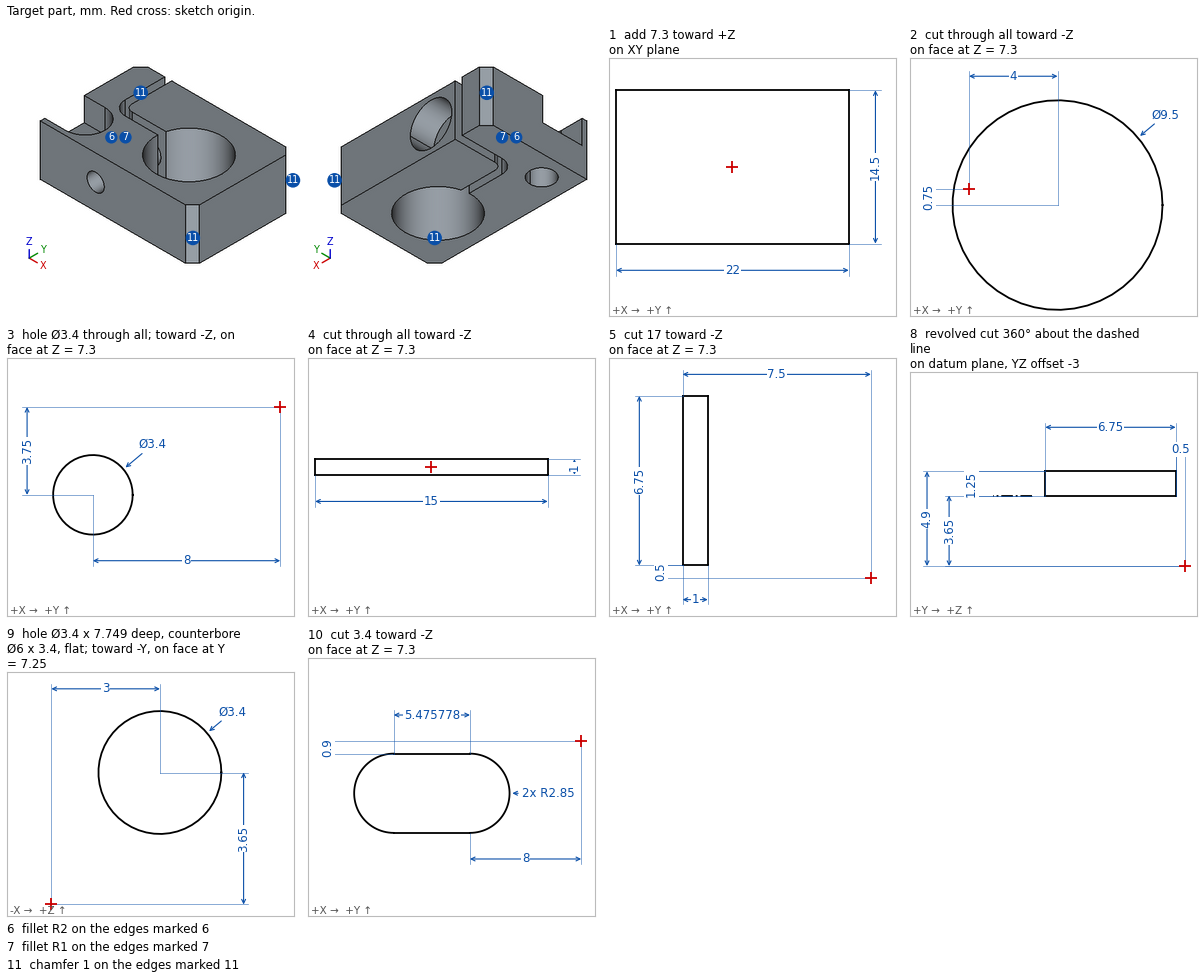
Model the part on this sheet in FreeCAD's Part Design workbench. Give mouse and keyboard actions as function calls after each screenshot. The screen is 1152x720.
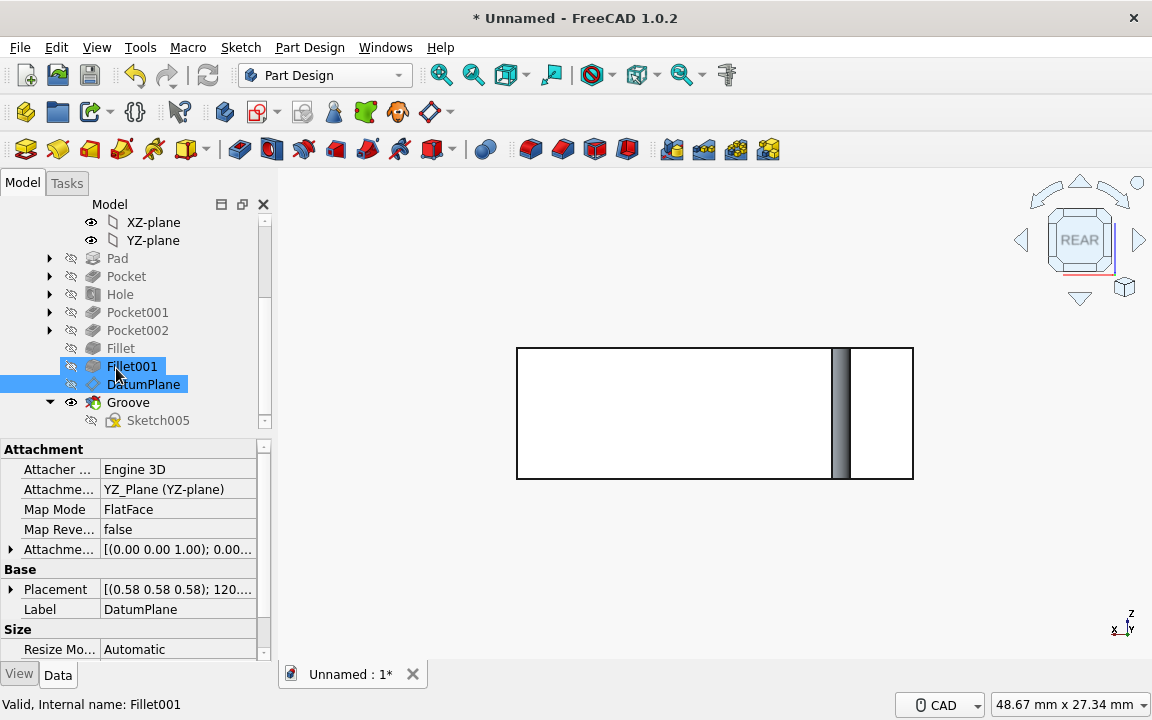
click(585, 412)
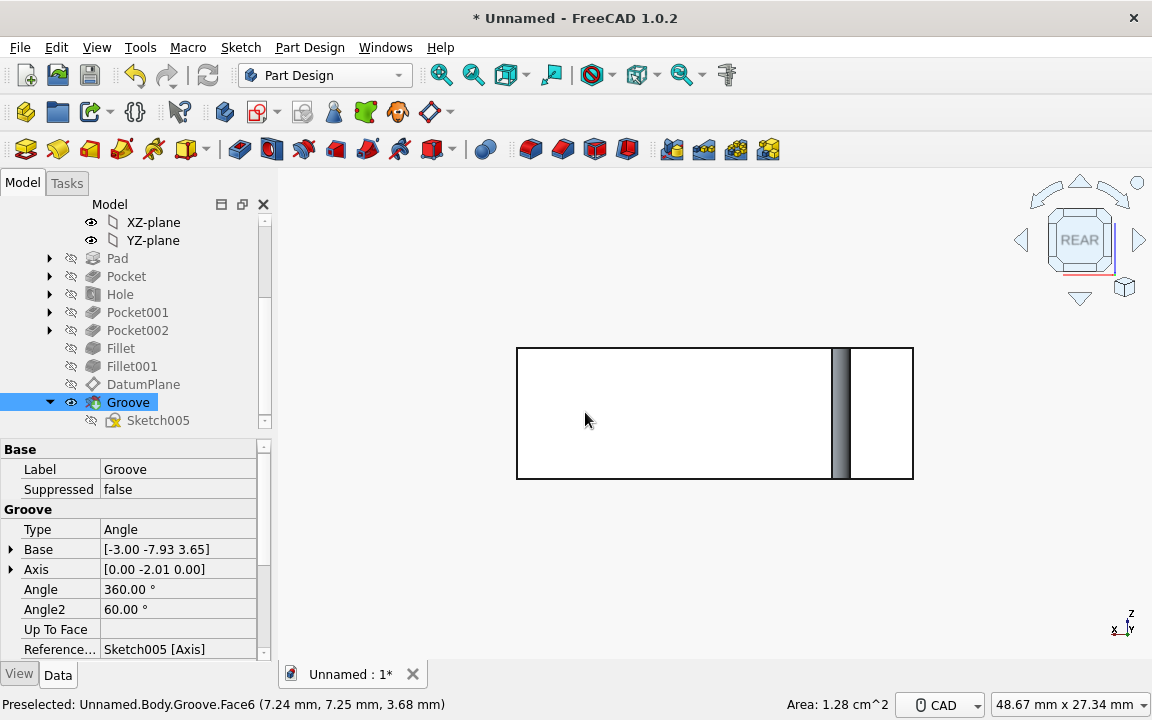
click(258, 112)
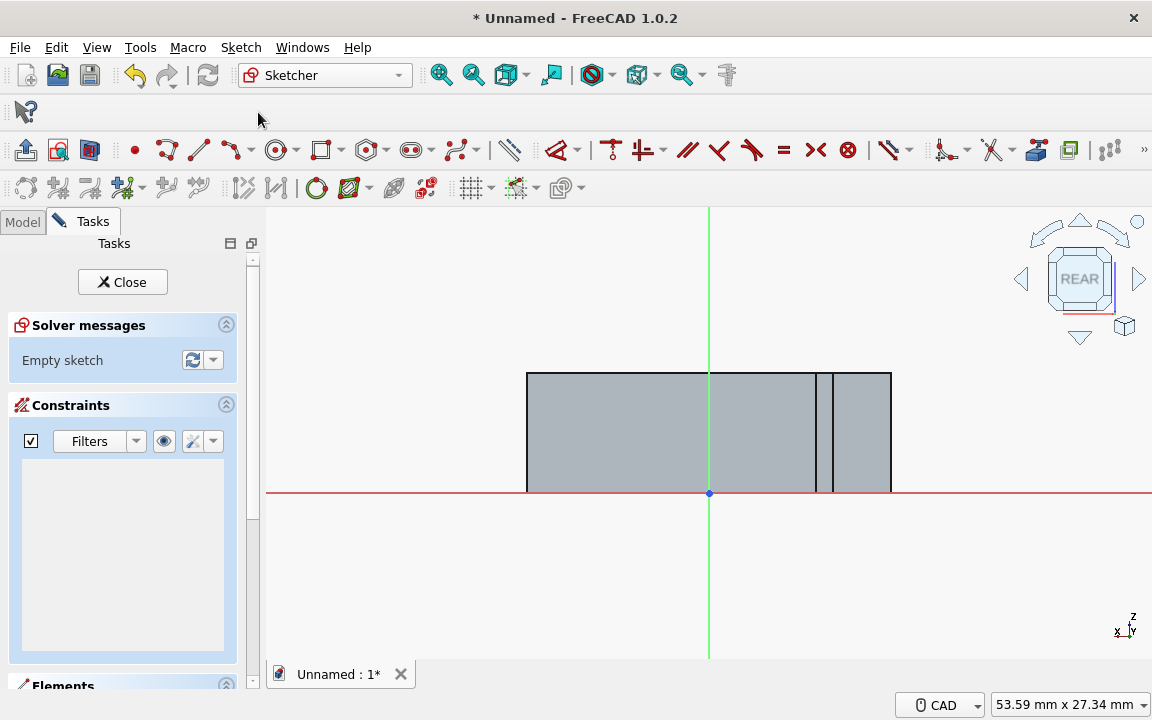
scroll(794, 456, up, 6)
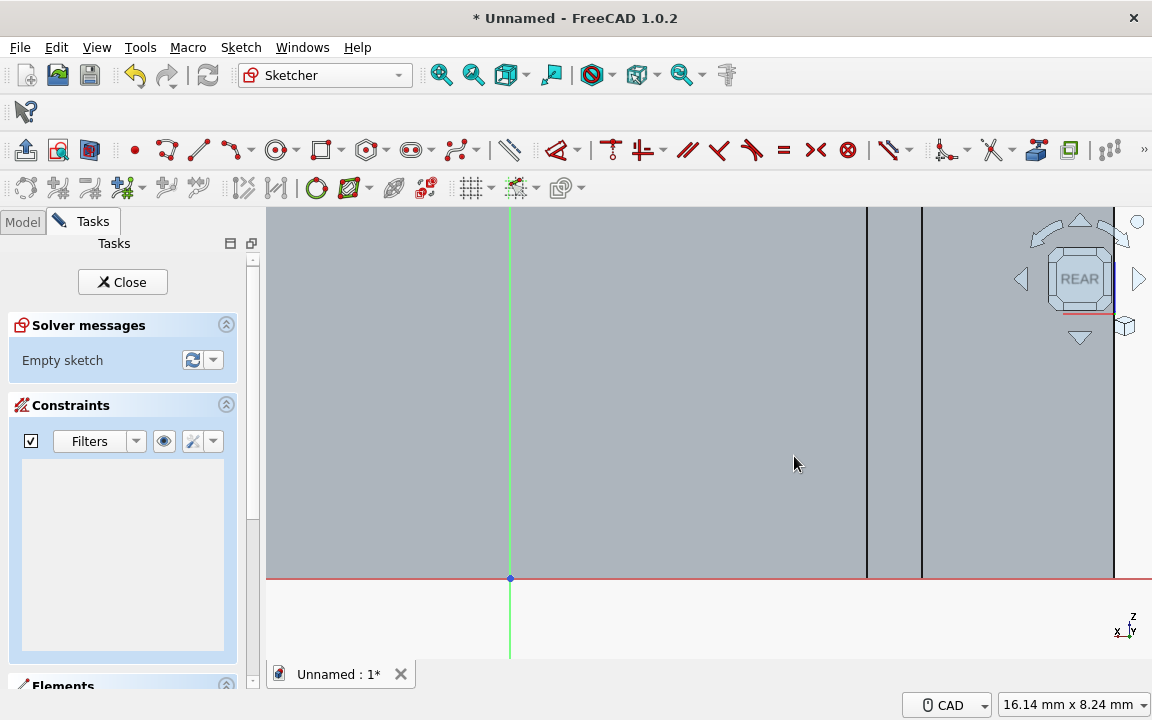
key(g)
key(c)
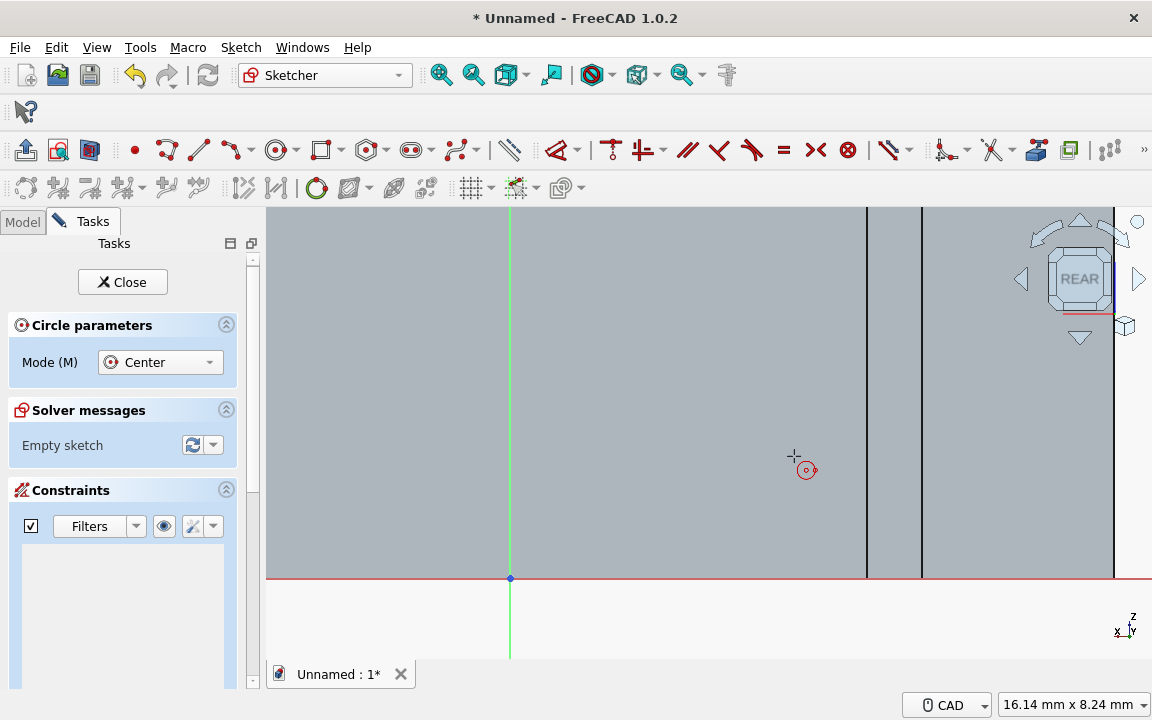
click(675, 378)
click(741, 312)
key(Escape)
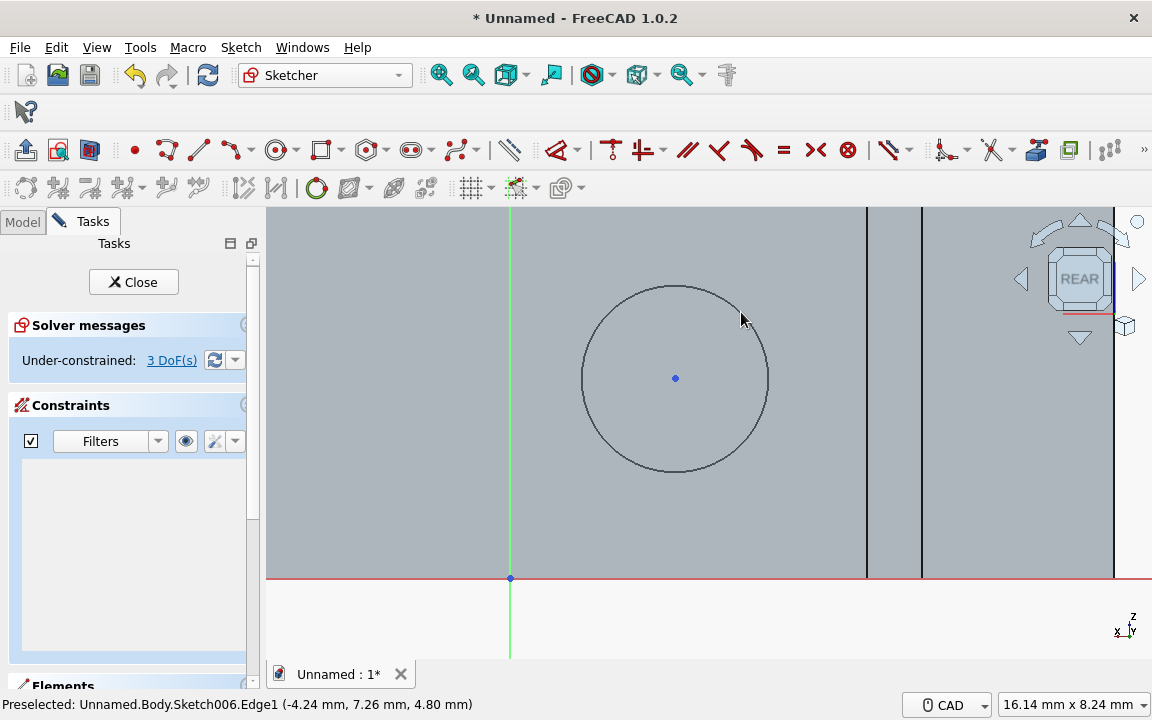
key(d)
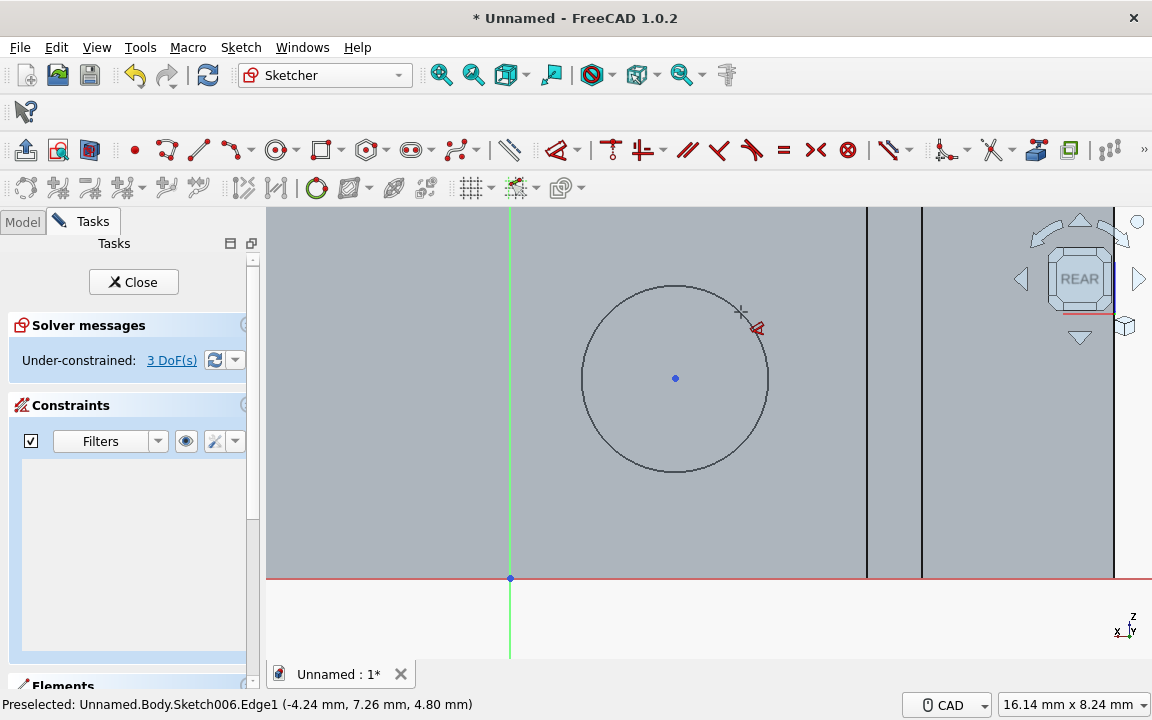
click(741, 313)
click(764, 290)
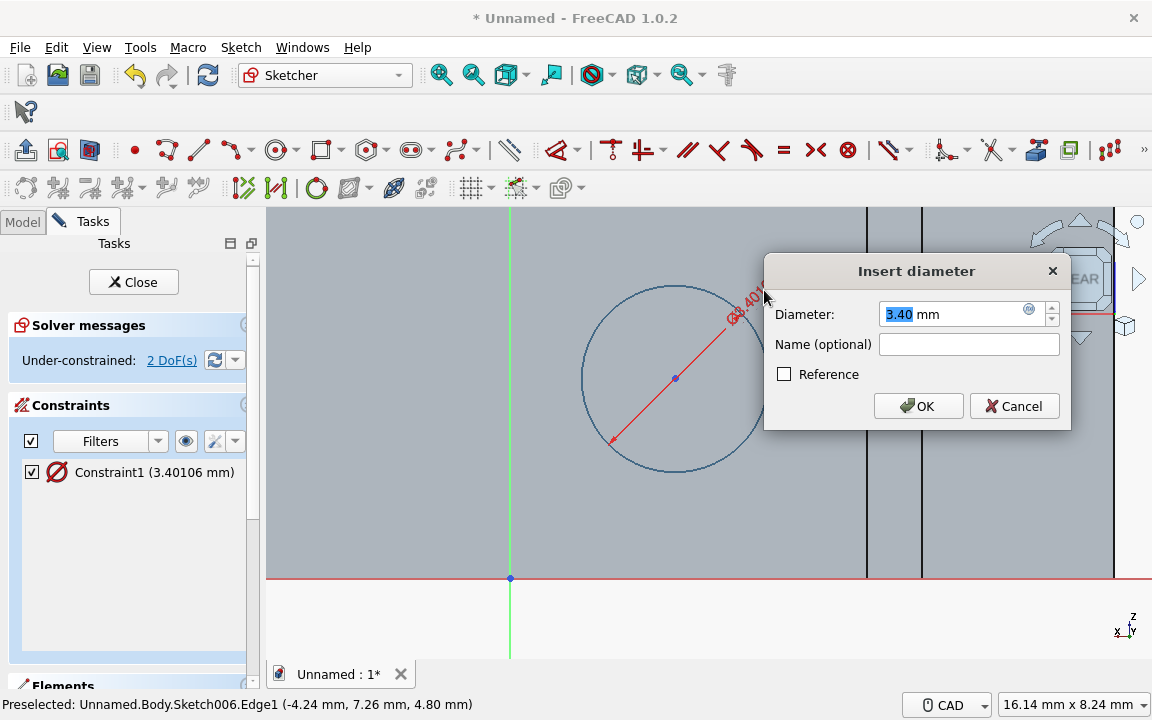
text(3.4)
key(Return)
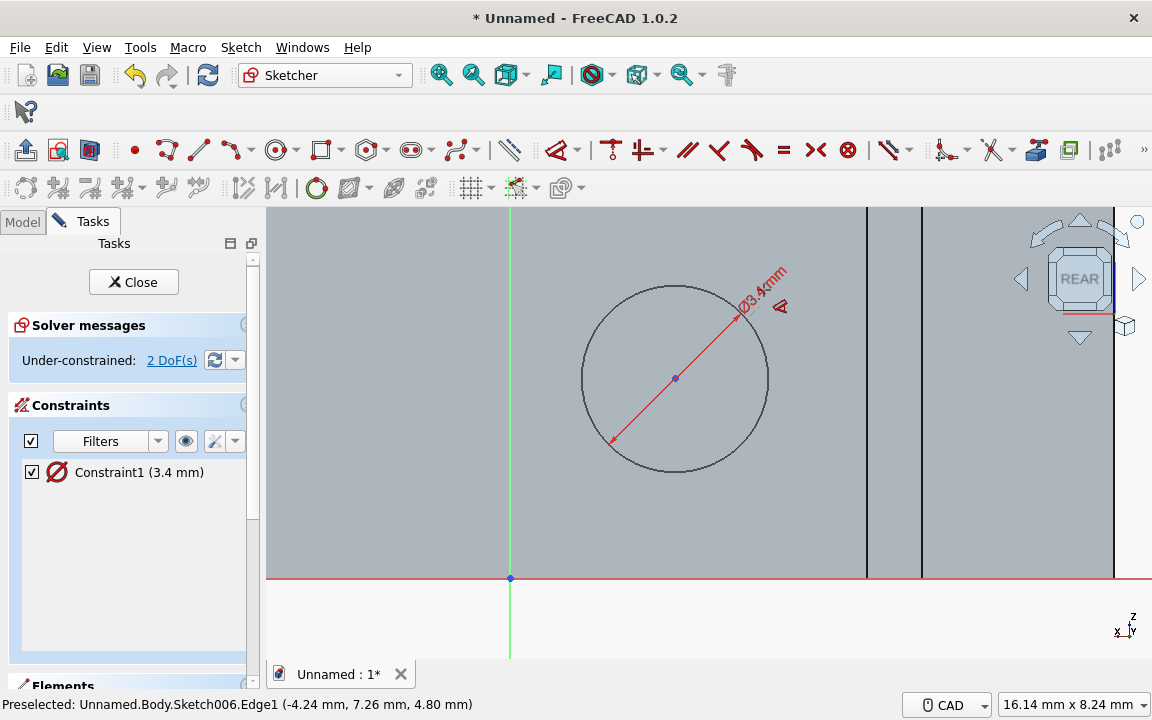
click(675, 379)
click(593, 613)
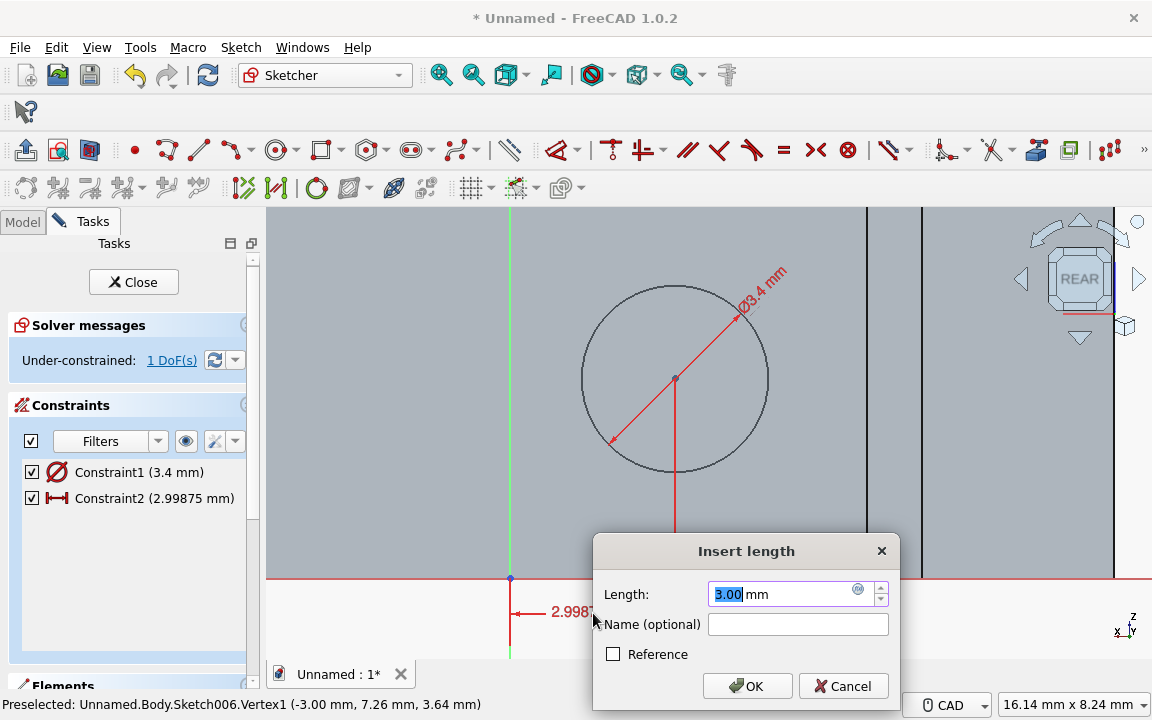
text(3)
key(Return)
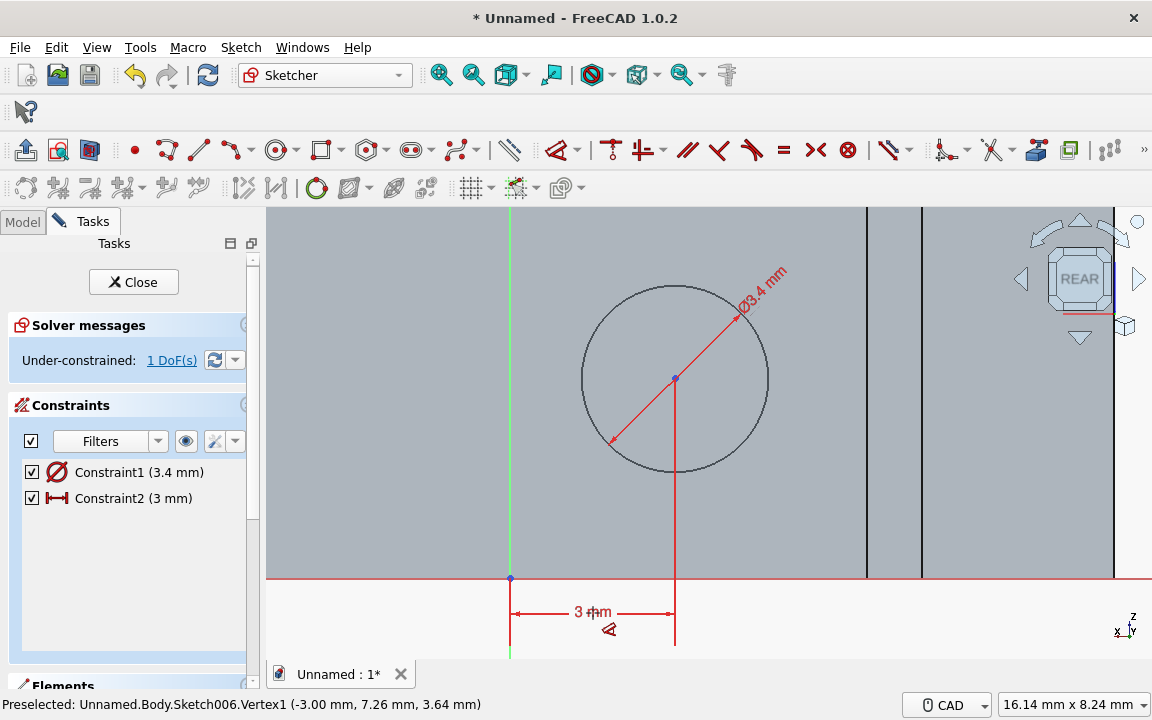
click(675, 379)
click(476, 479)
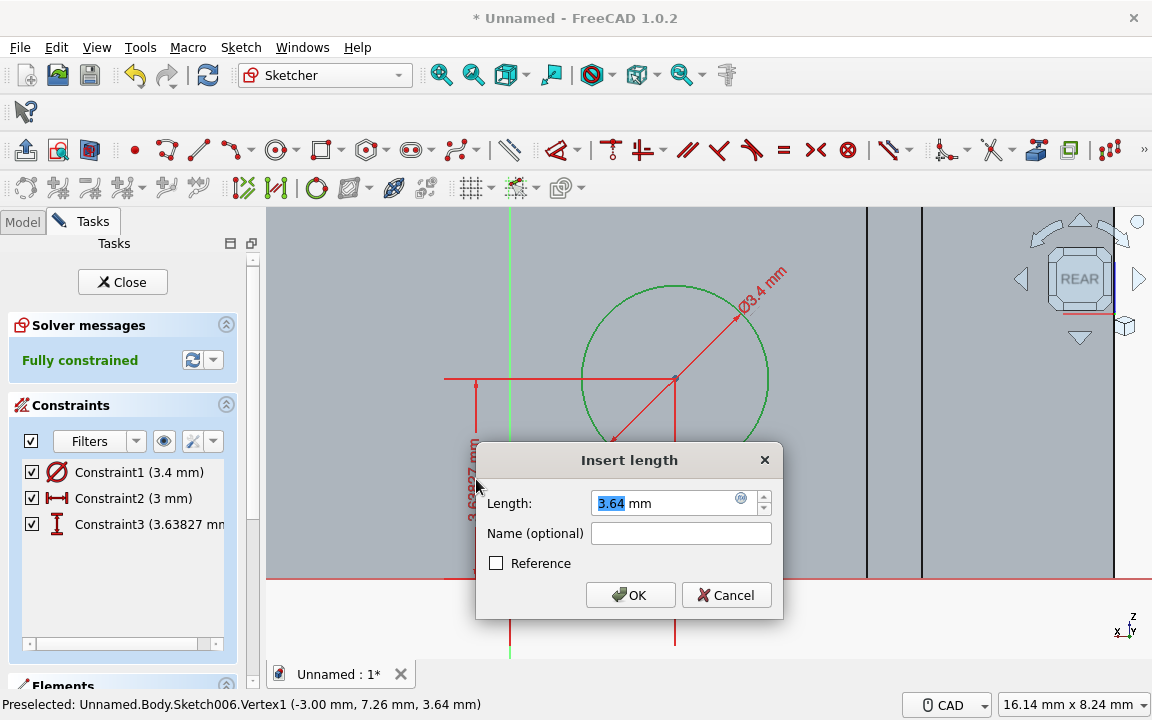
text(3.65)
key(Return)
key(Escape)